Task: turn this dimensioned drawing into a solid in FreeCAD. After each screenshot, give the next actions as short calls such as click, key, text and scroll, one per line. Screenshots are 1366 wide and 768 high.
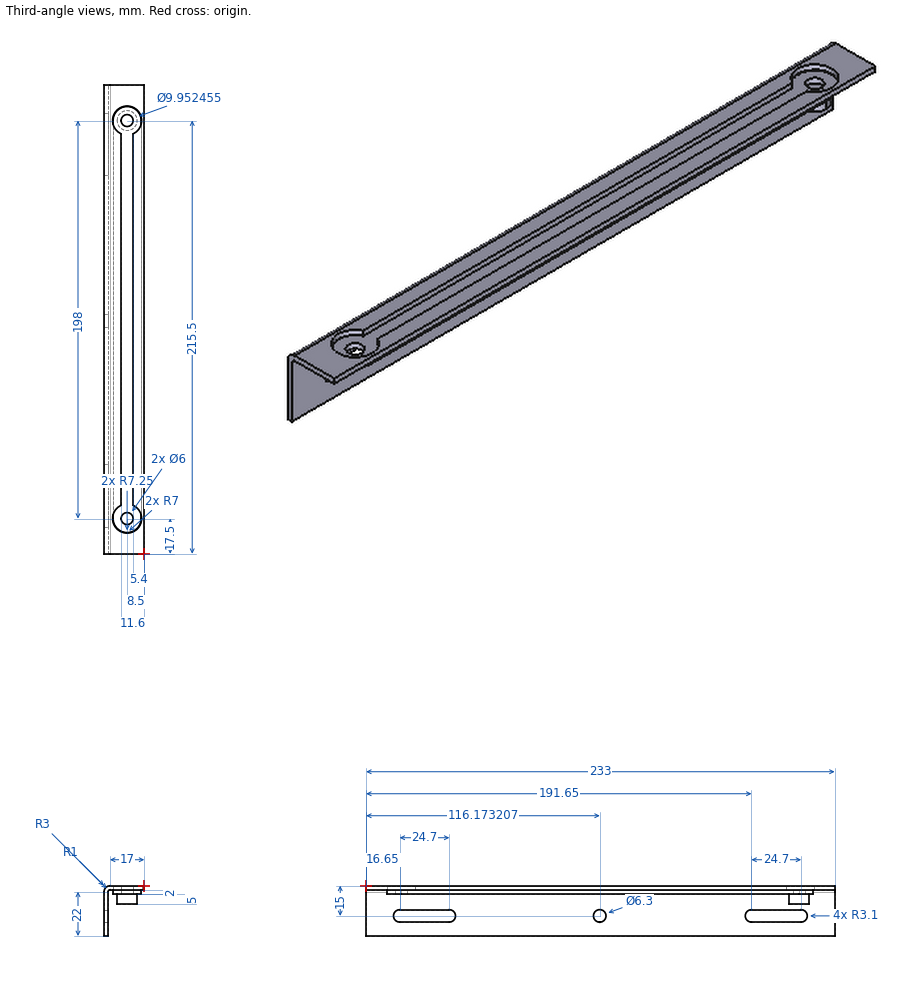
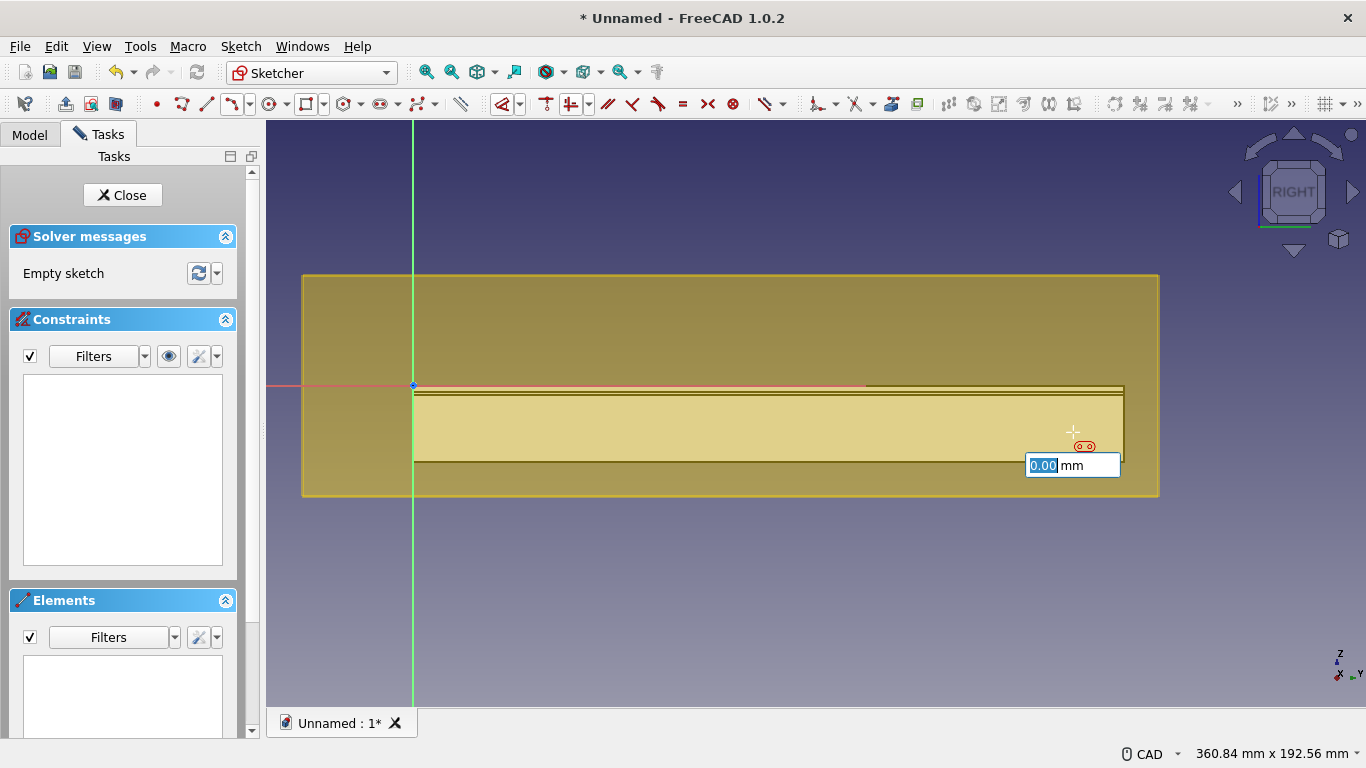
scroll(1035, 441, up, 3)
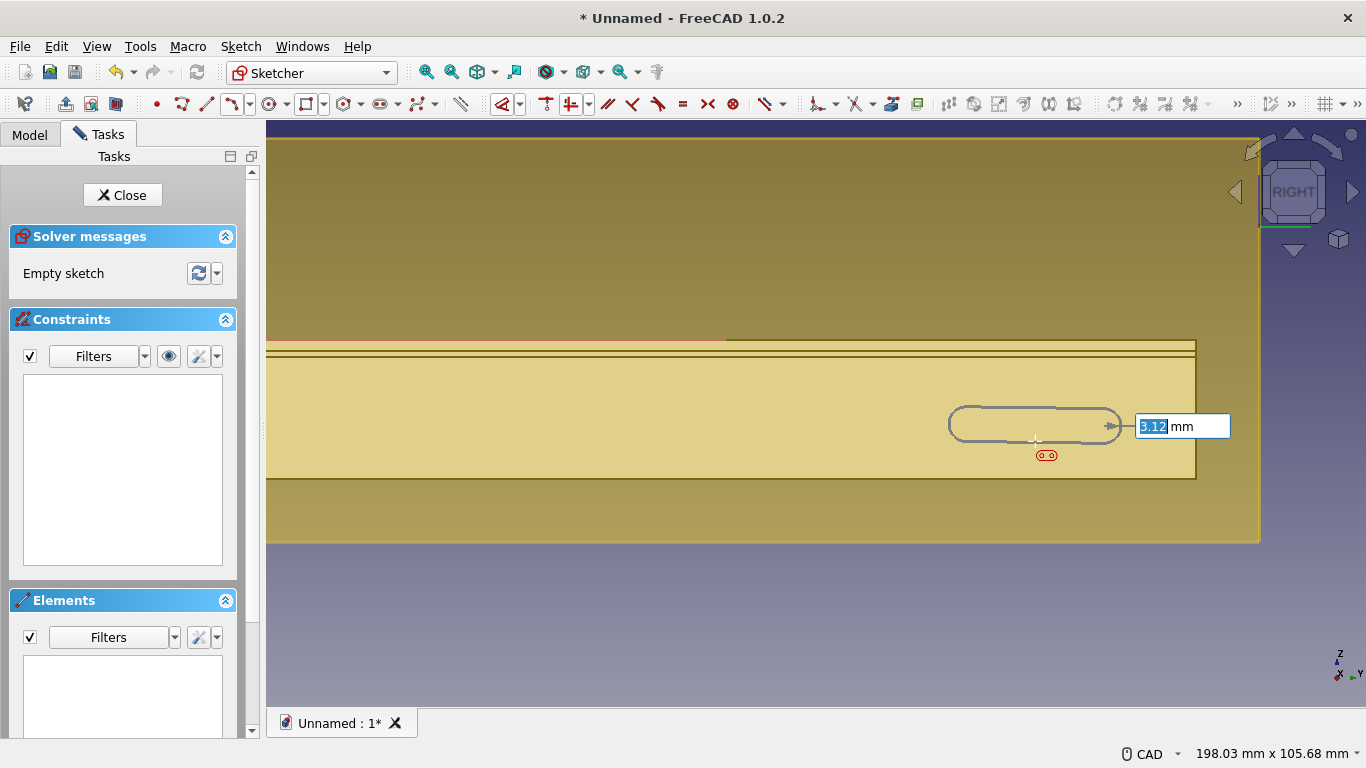
click(1035, 441)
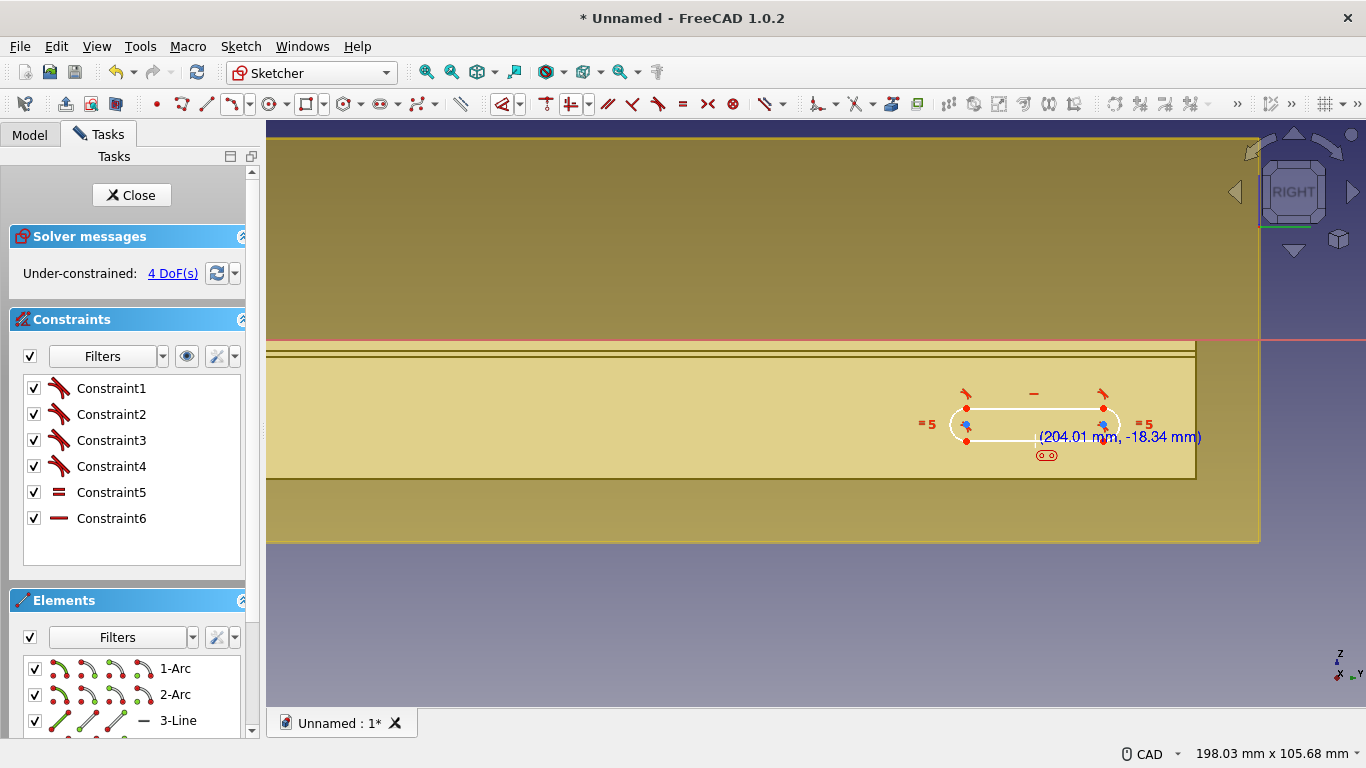
scroll(1035, 441, down, 3)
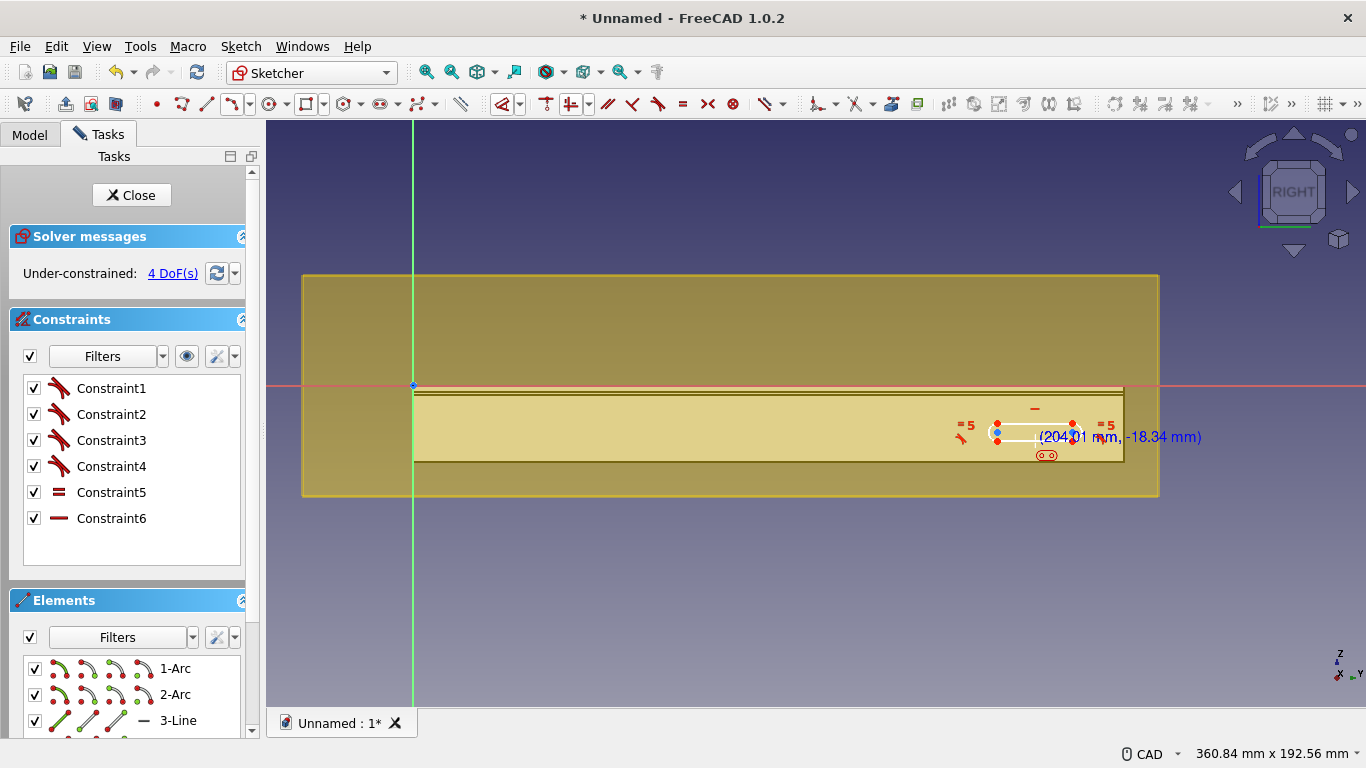
scroll(464, 432, up, 5)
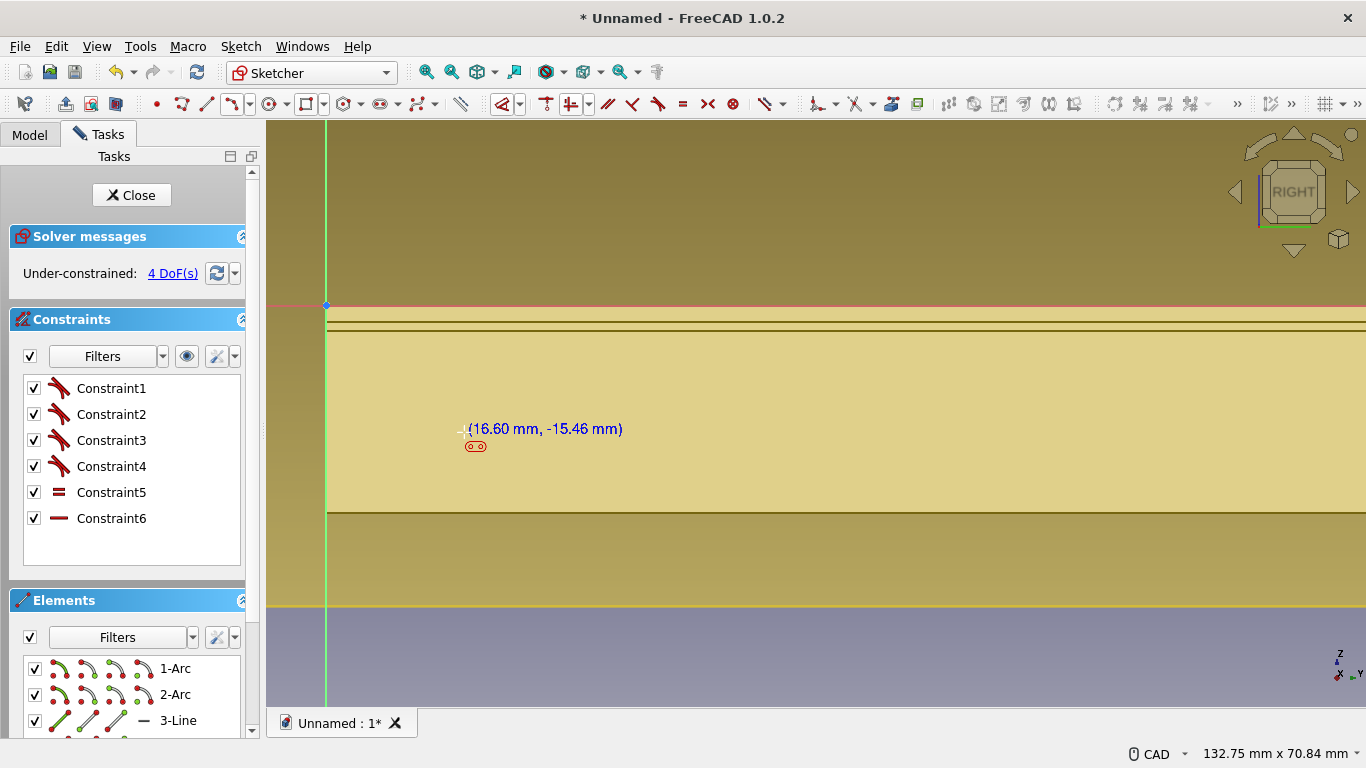
click(464, 430)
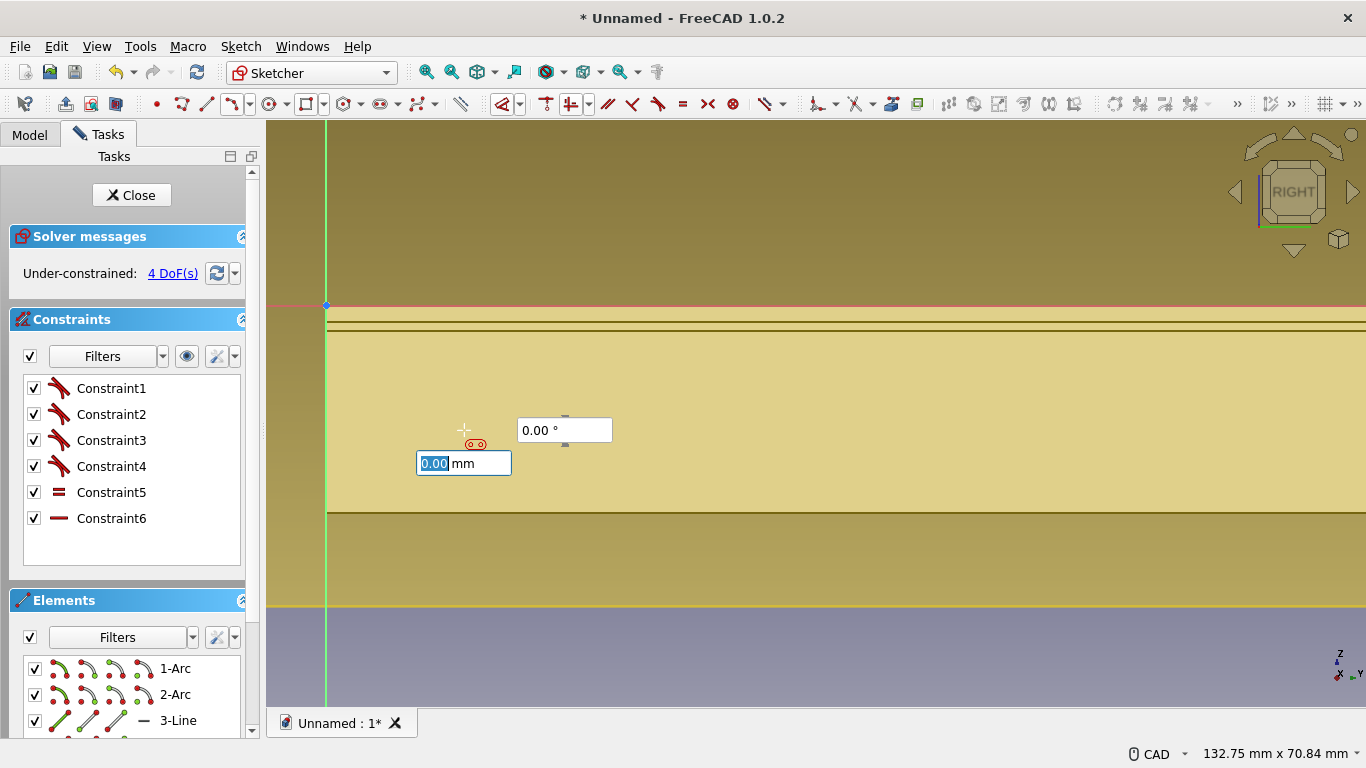
click(669, 430)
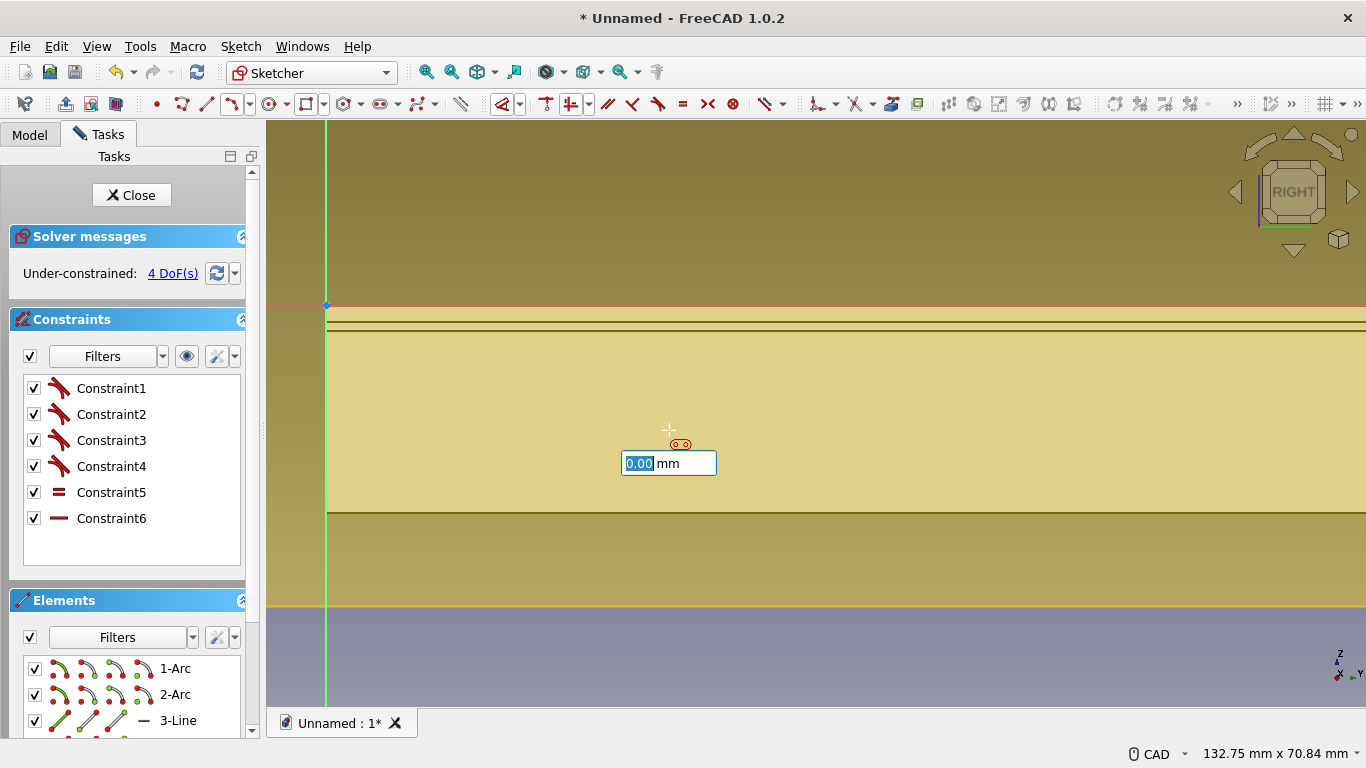
click(566, 456)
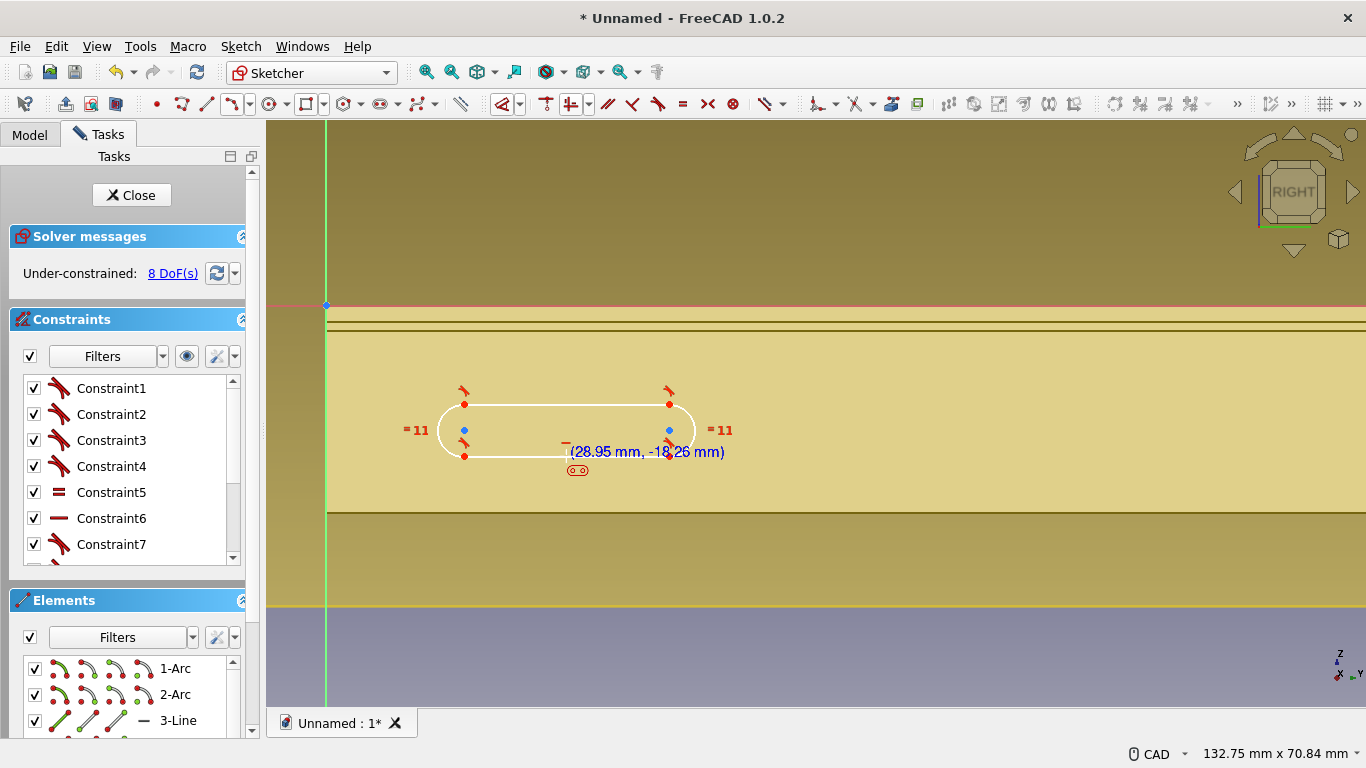
click(268, 104)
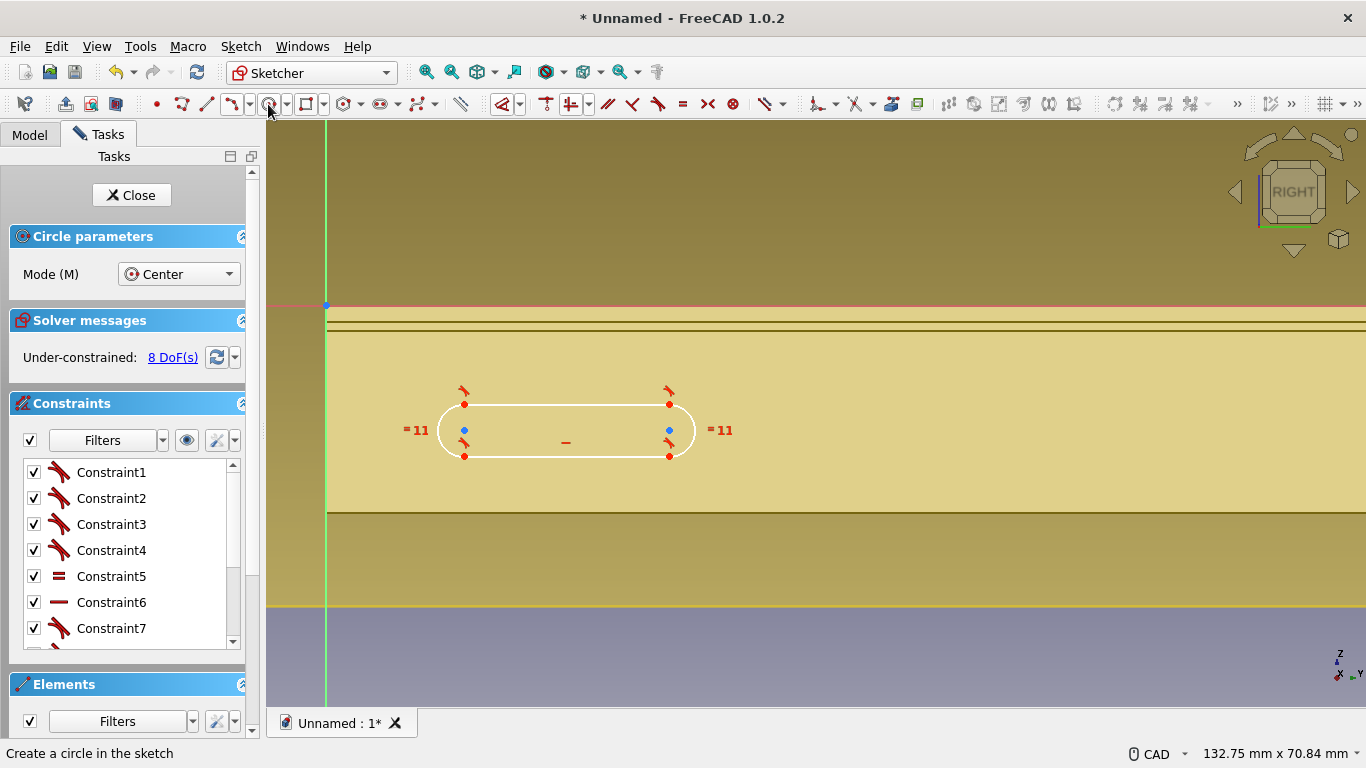
scroll(464, 432, down, 5)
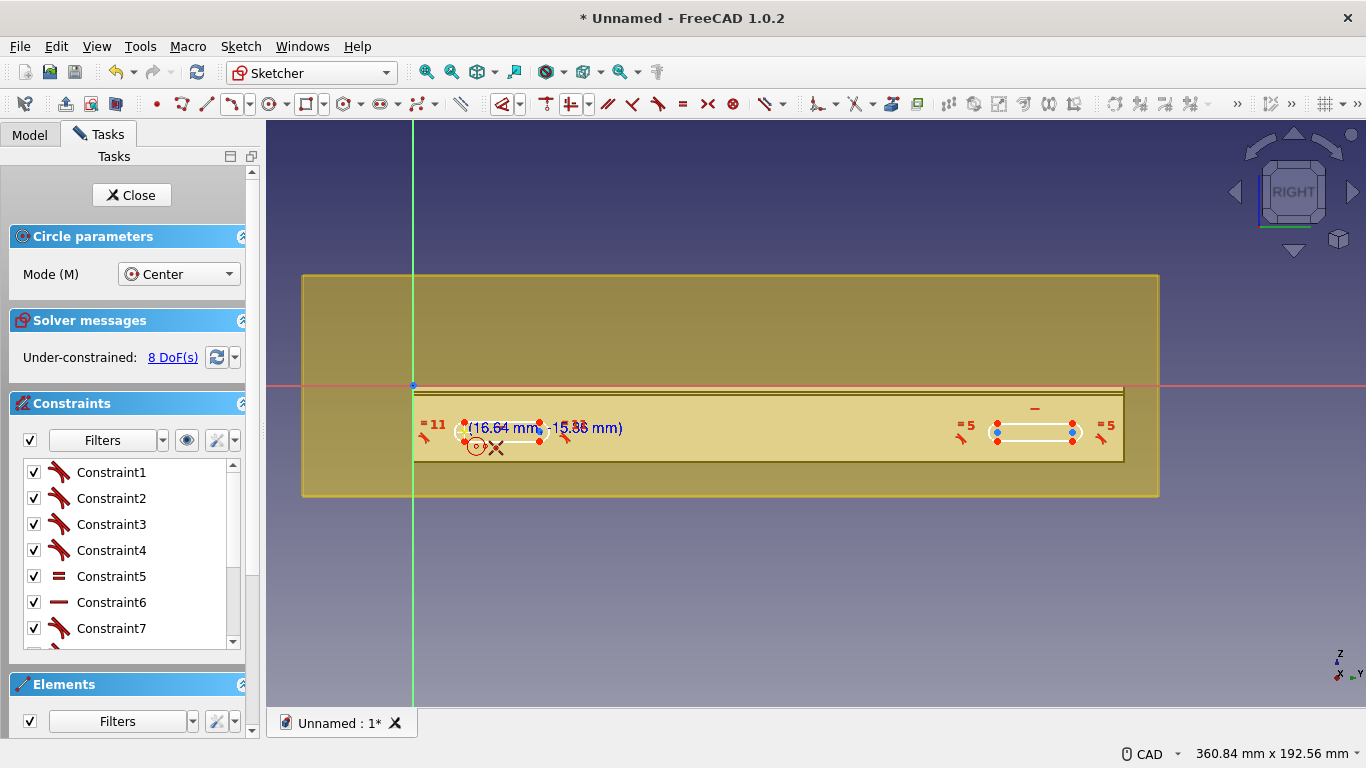
scroll(768, 432, up, 5)